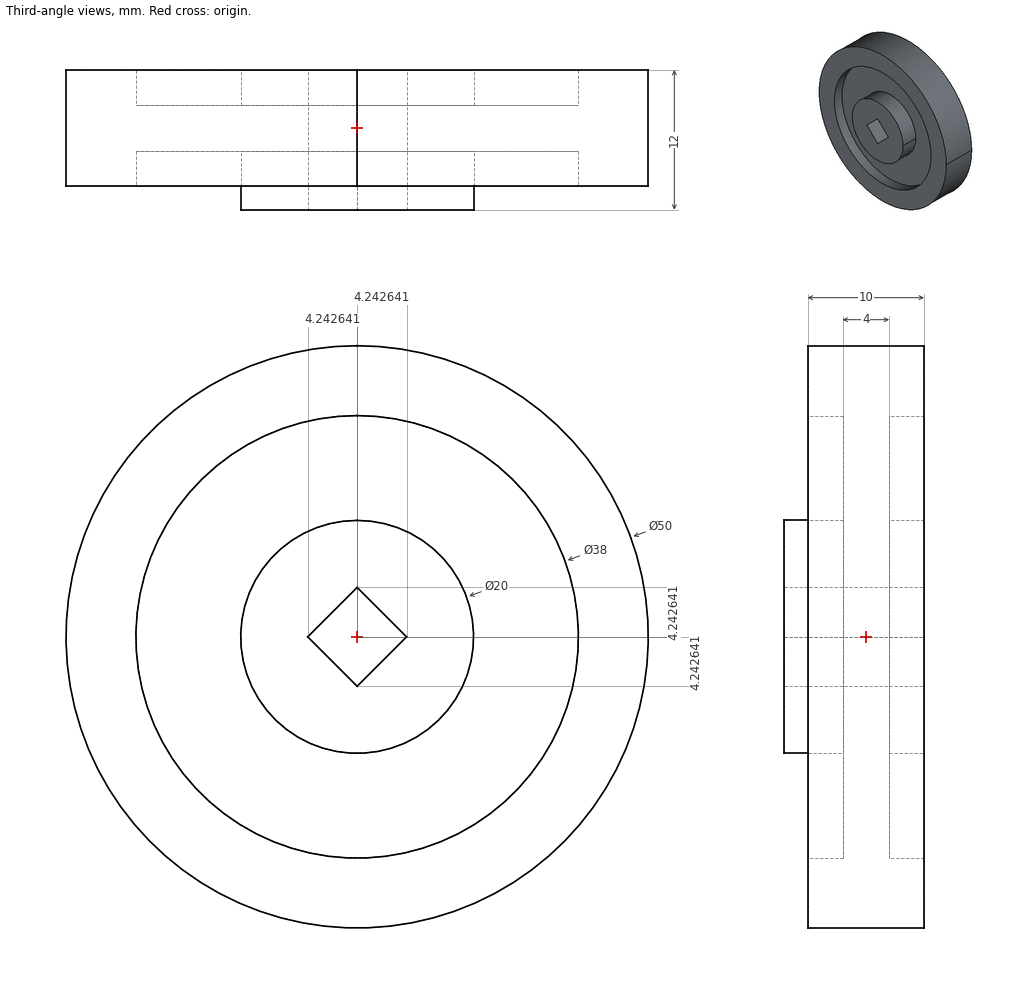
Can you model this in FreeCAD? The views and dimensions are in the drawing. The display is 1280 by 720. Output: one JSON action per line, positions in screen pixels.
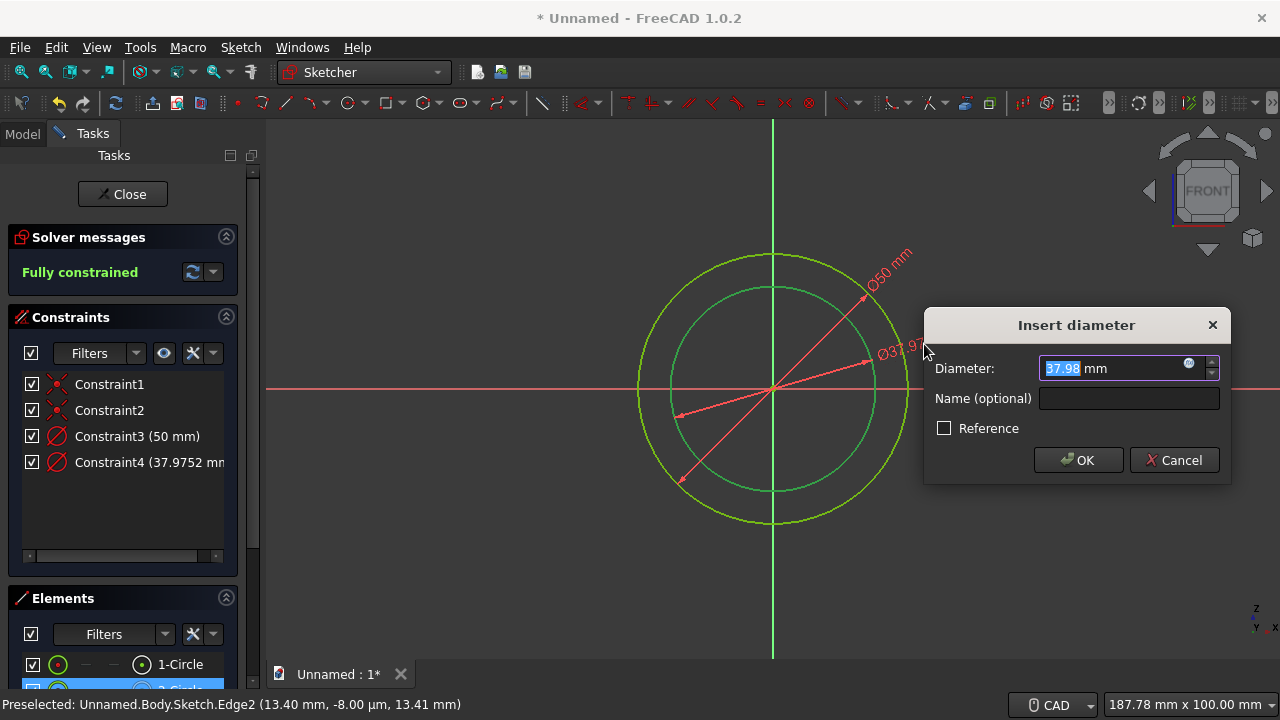
{"action": "type", "text": "38"}
{"action": "key", "text": "Return"}
{"action": "key", "text": "Escape"}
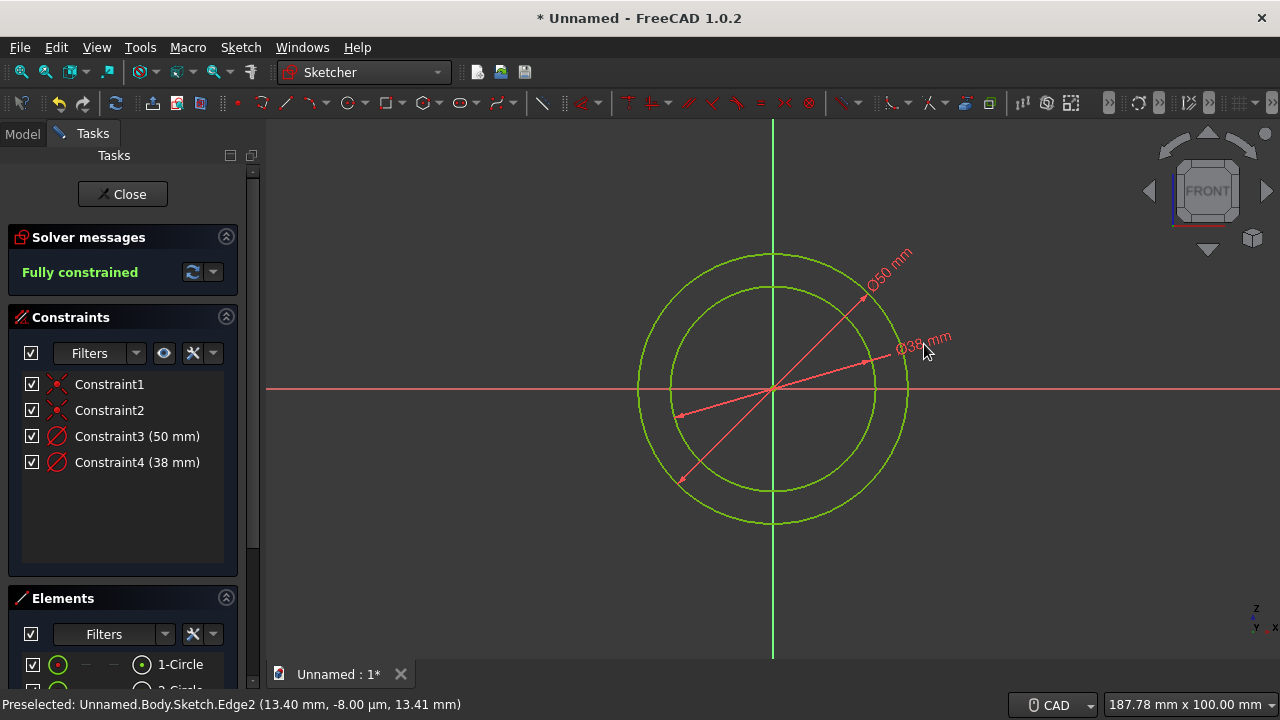
{"action": "left_click", "coordinate": [123, 194]}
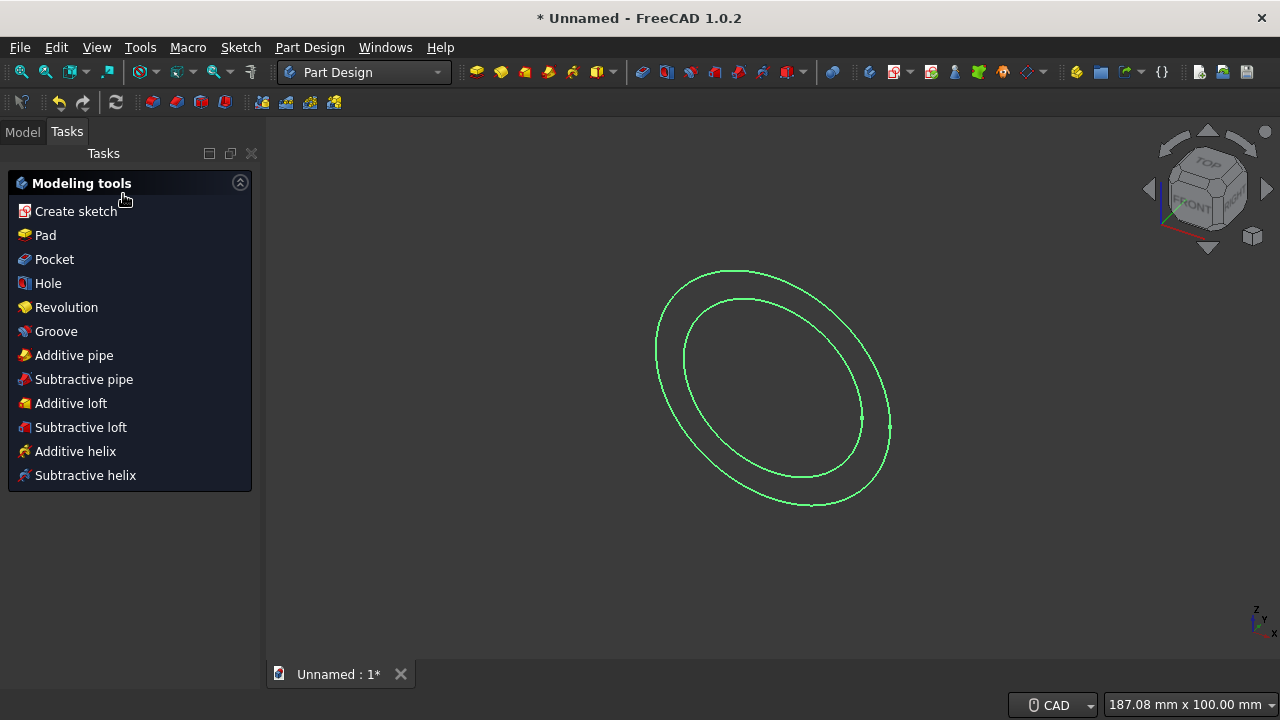
{"action": "left_click", "coordinate": [478, 72]}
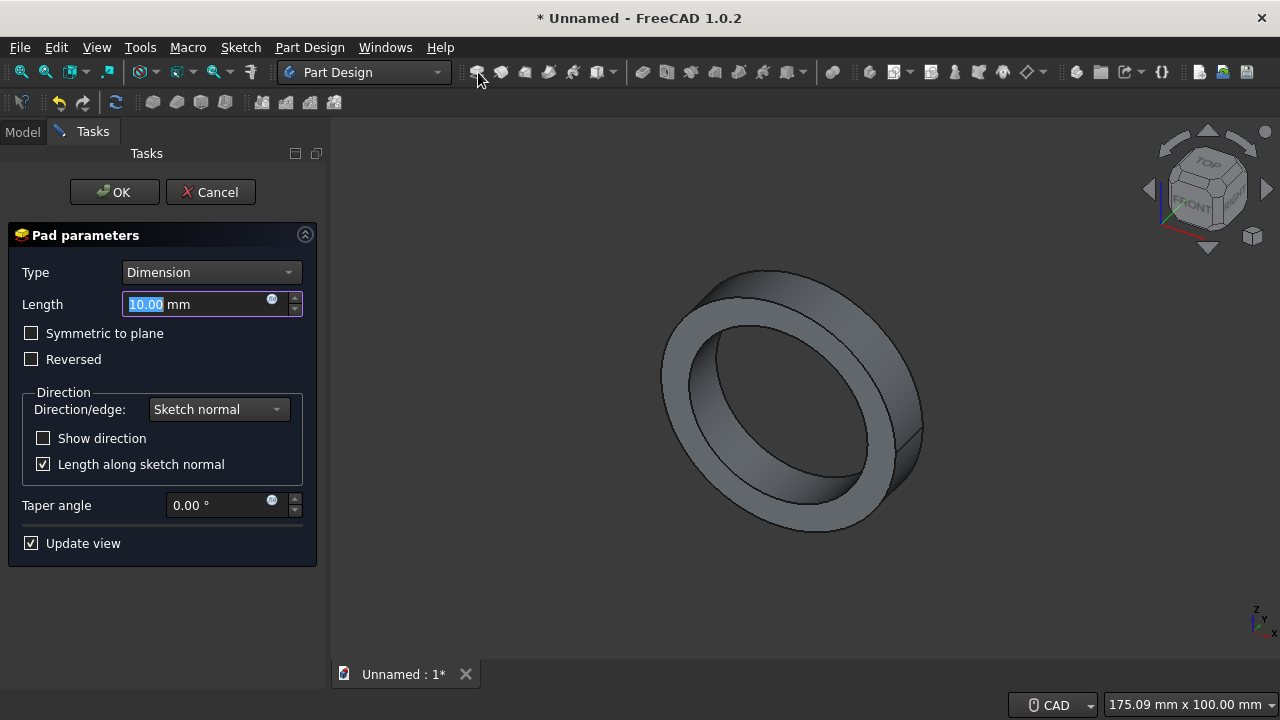
{"action": "type", "text": "10"}
{"action": "key", "text": "Tab"}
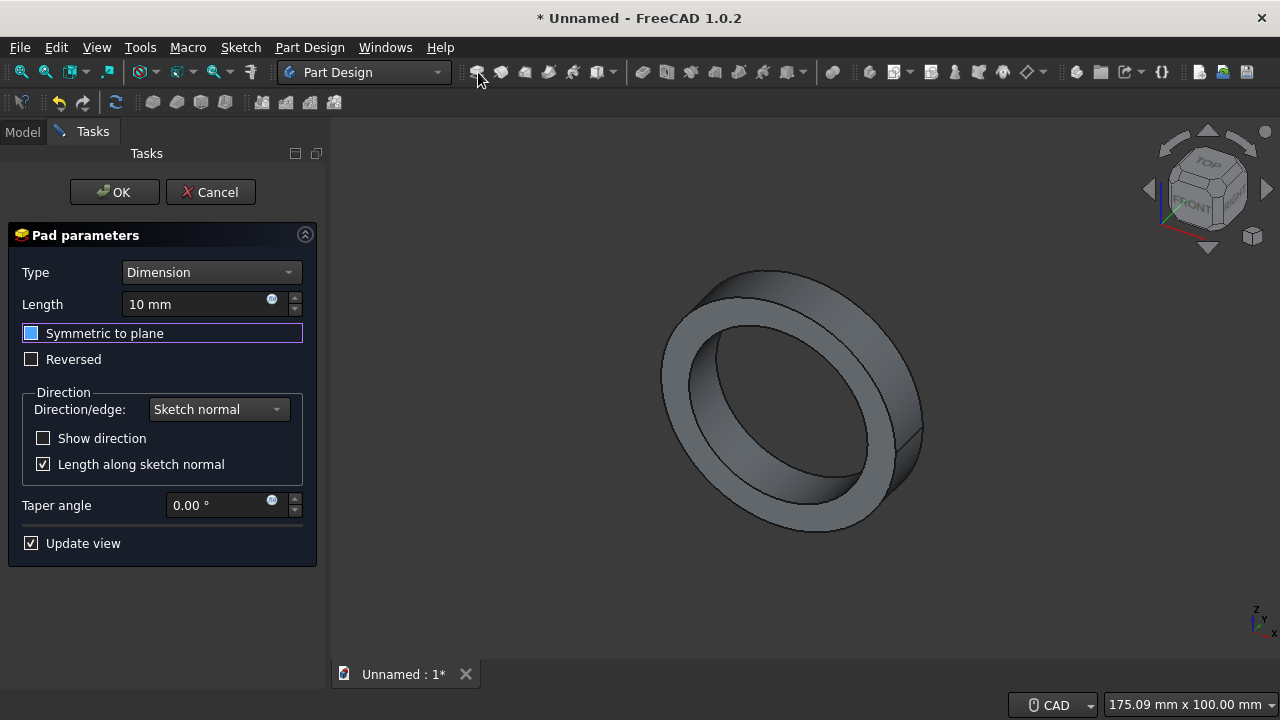
{"action": "left_click", "coordinate": [30, 333]}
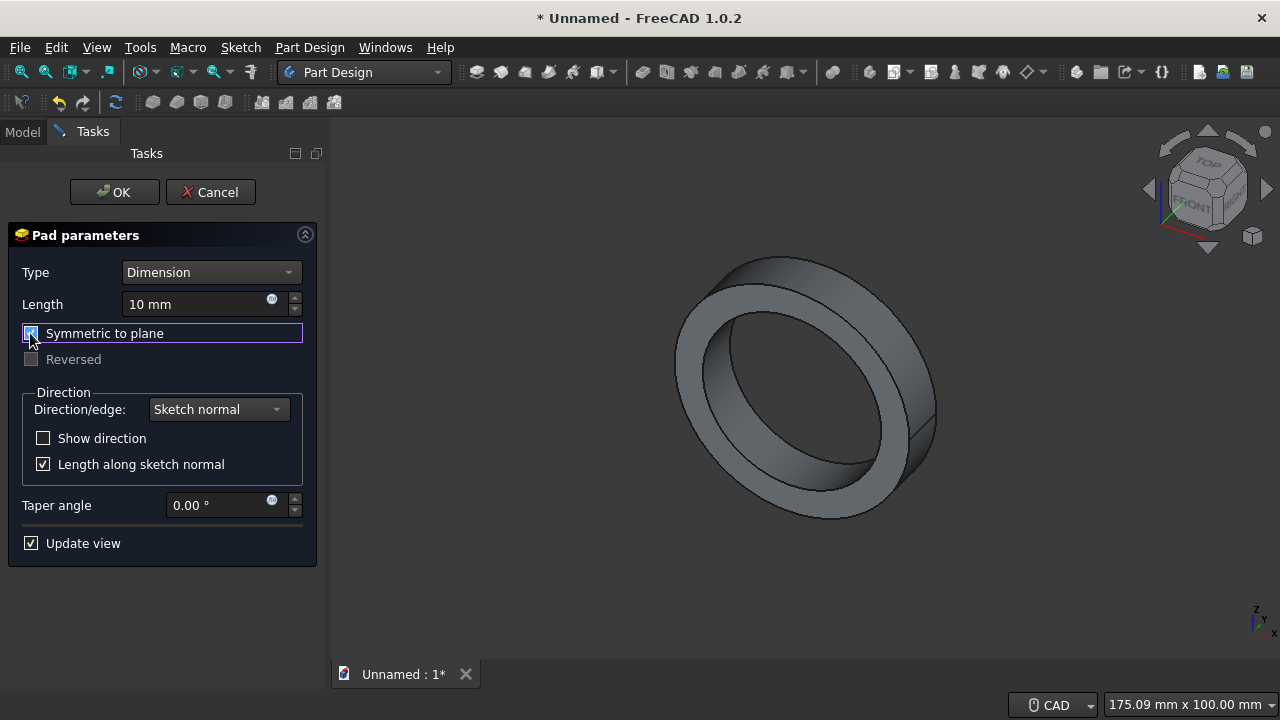
{"action": "left_click", "coordinate": [115, 192]}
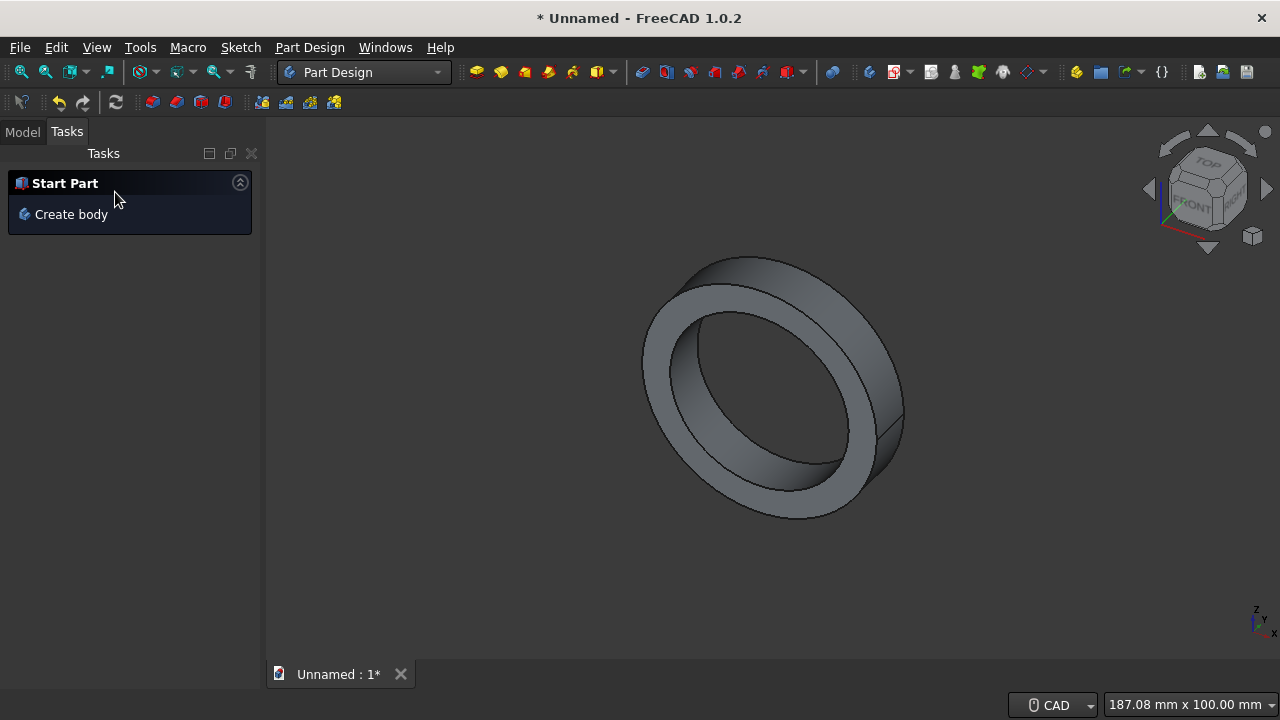
{"action": "left_click", "coordinate": [870, 72]}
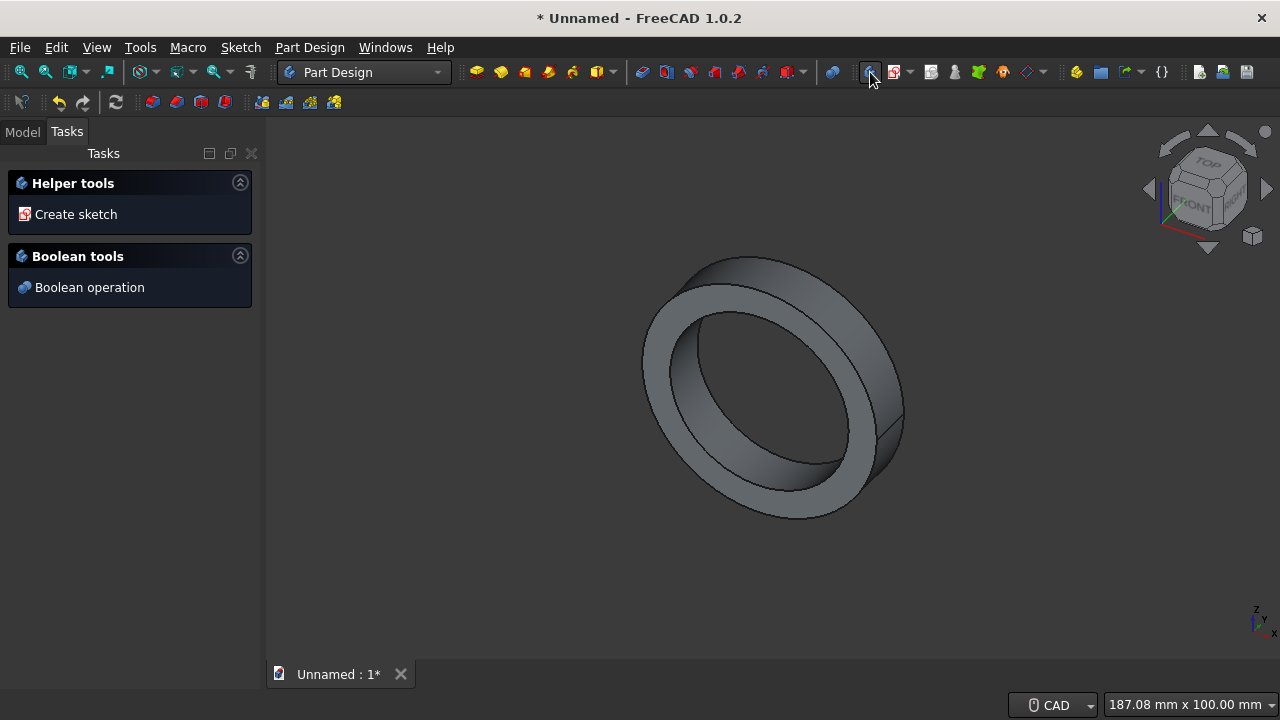
{"action": "left_click", "coordinate": [23, 131]}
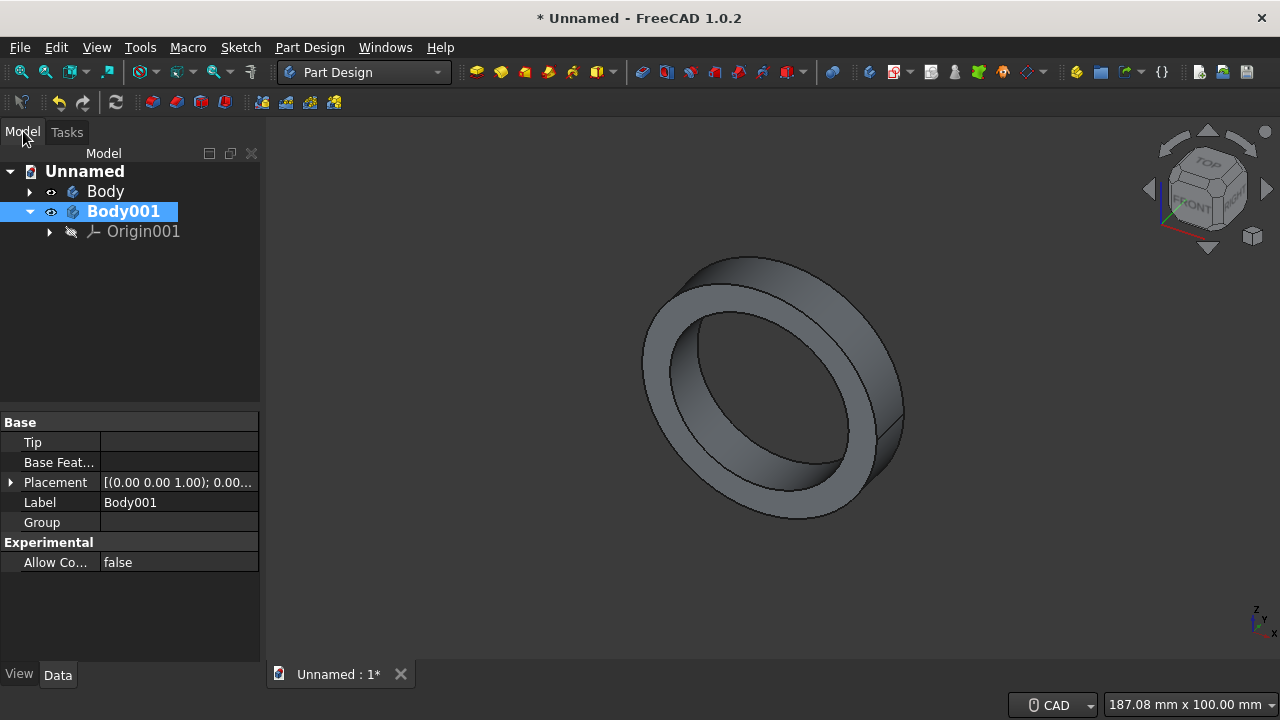
{"action": "left_click", "coordinate": [50, 232]}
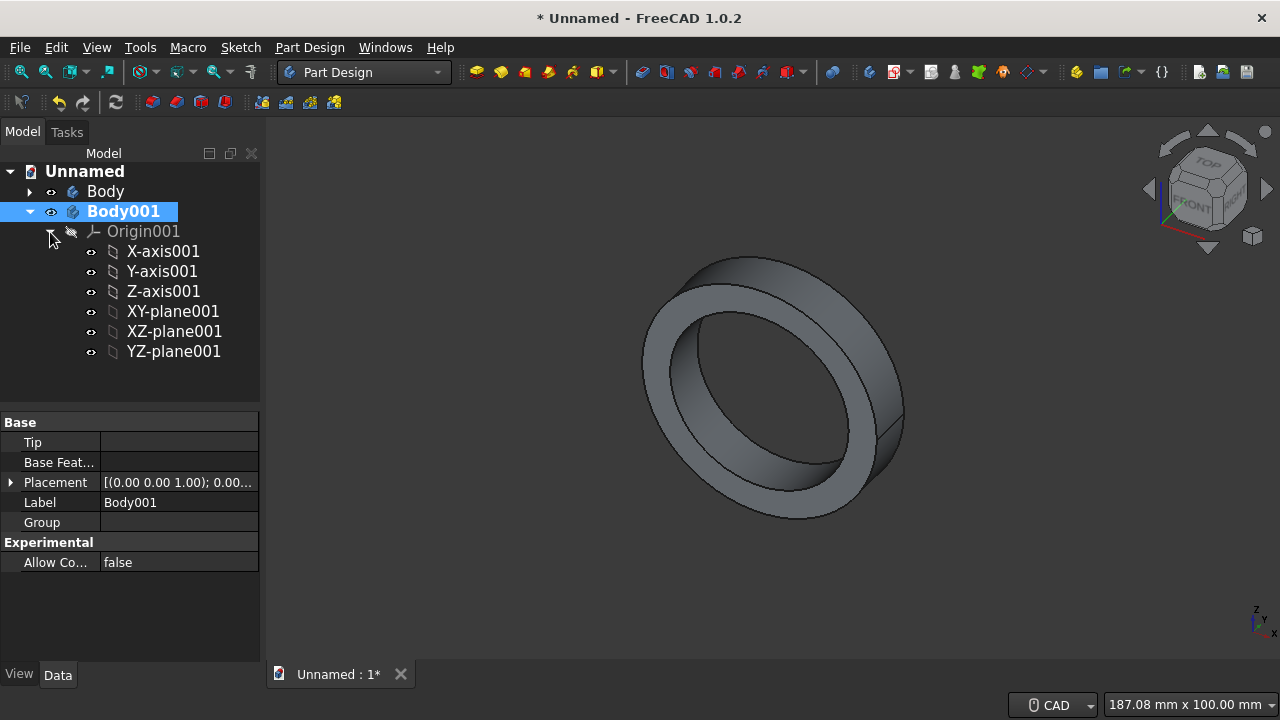
{"action": "left_click", "coordinate": [136, 332]}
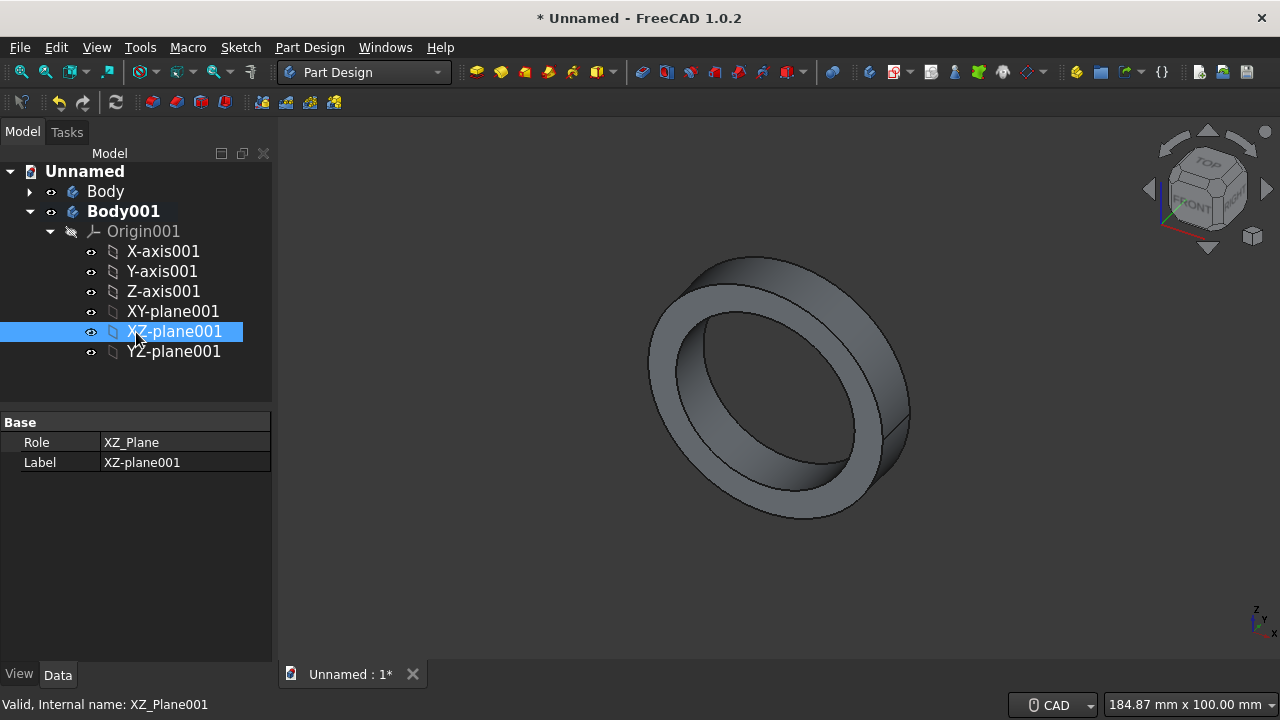
{"action": "left_click", "coordinate": [1028, 72]}